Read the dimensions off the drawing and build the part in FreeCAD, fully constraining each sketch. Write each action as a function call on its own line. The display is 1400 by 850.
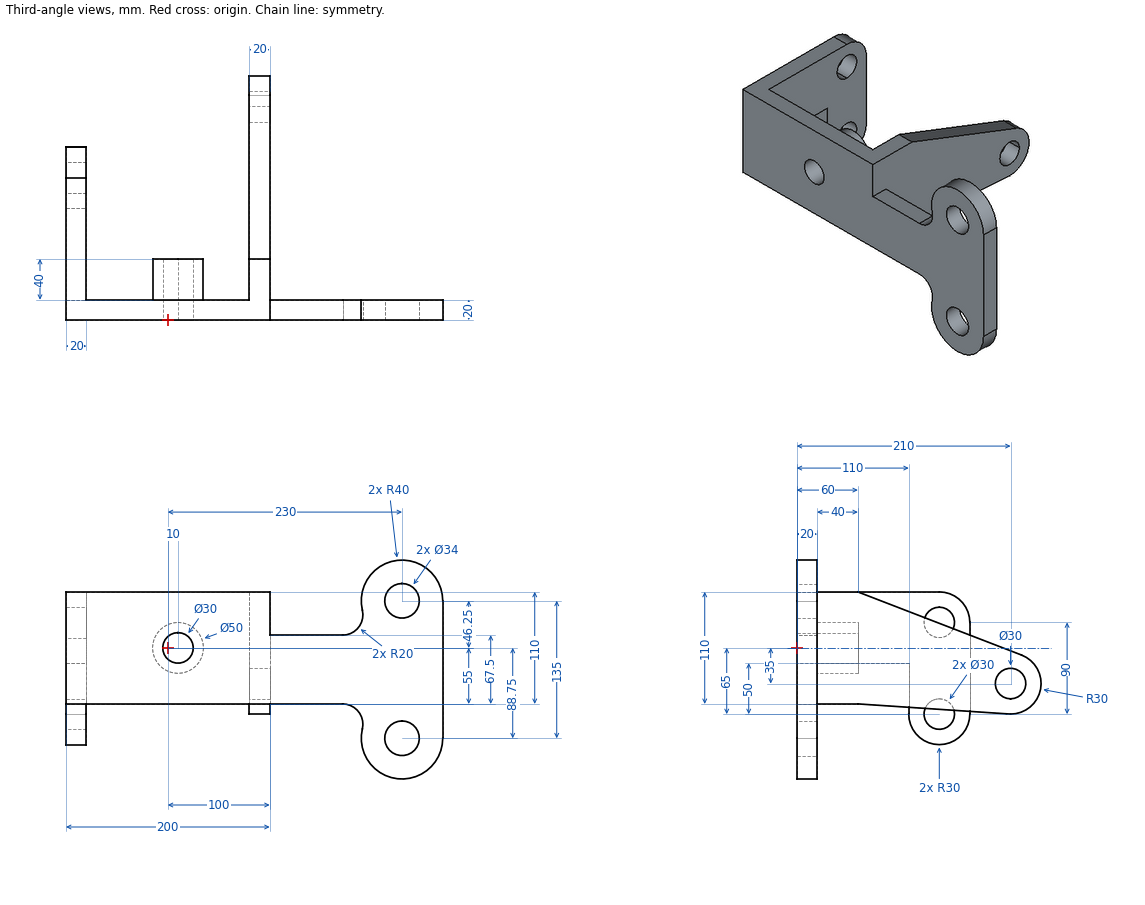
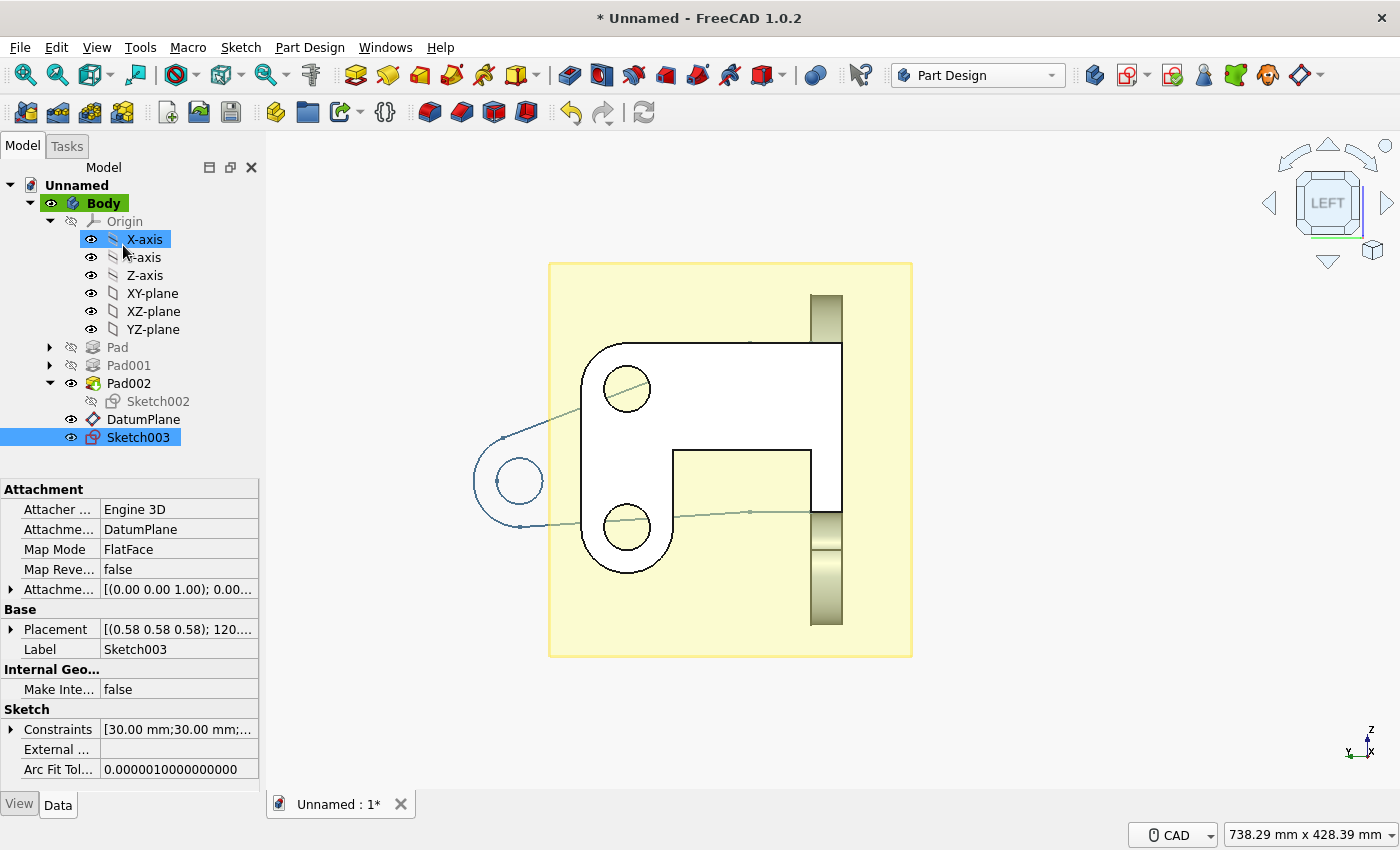
click(356, 76)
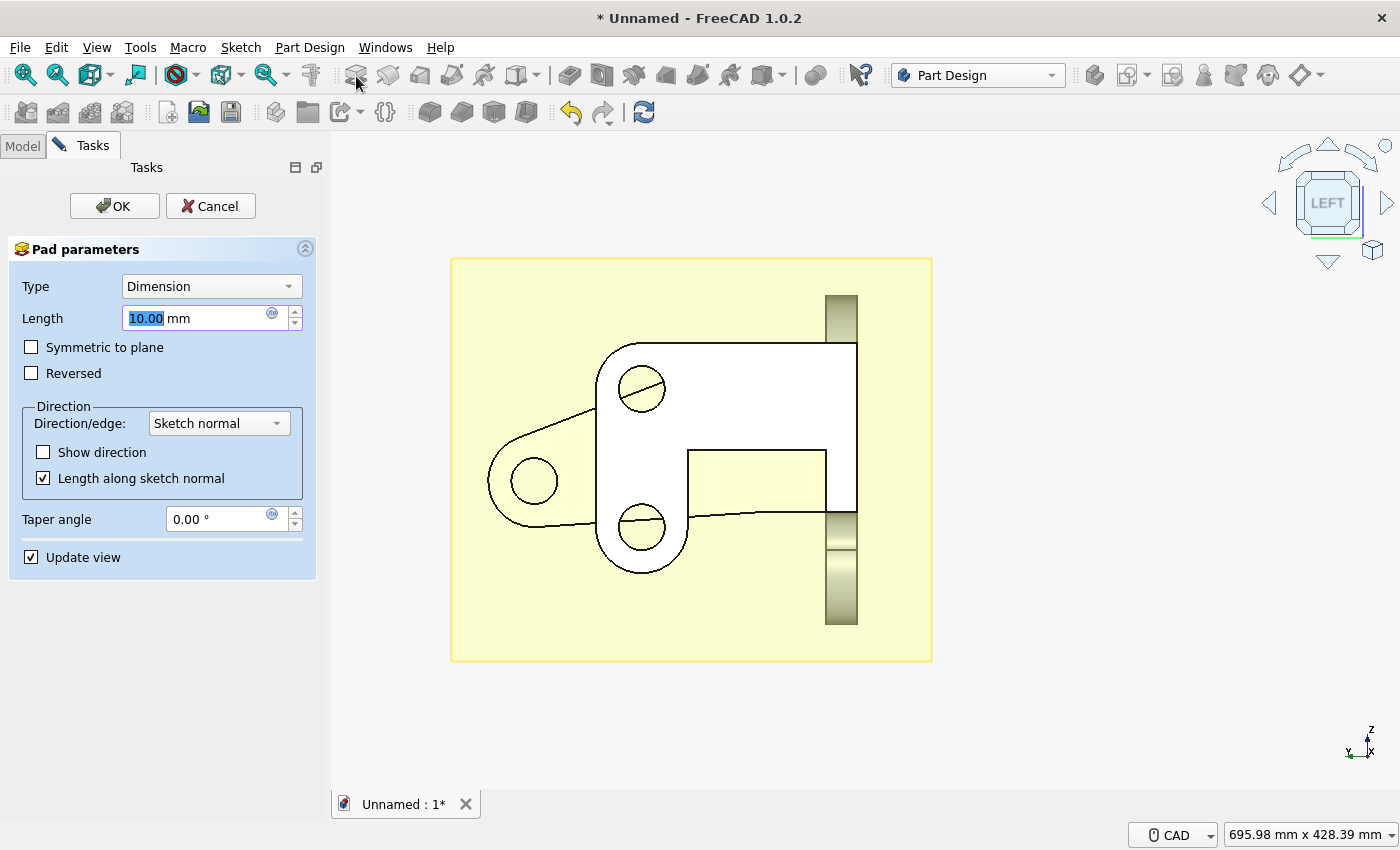
text(20)
key(Tab)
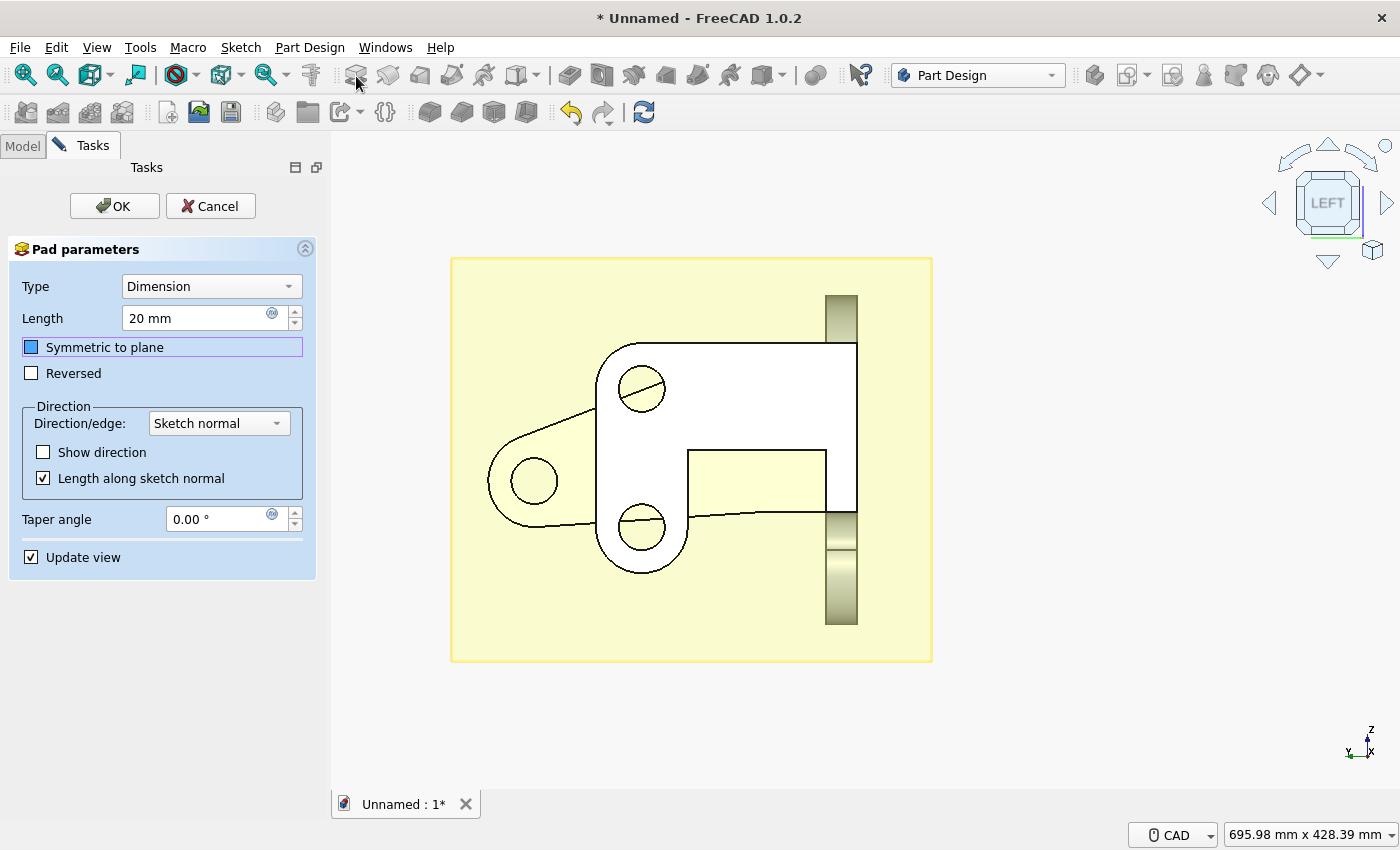
click(30, 373)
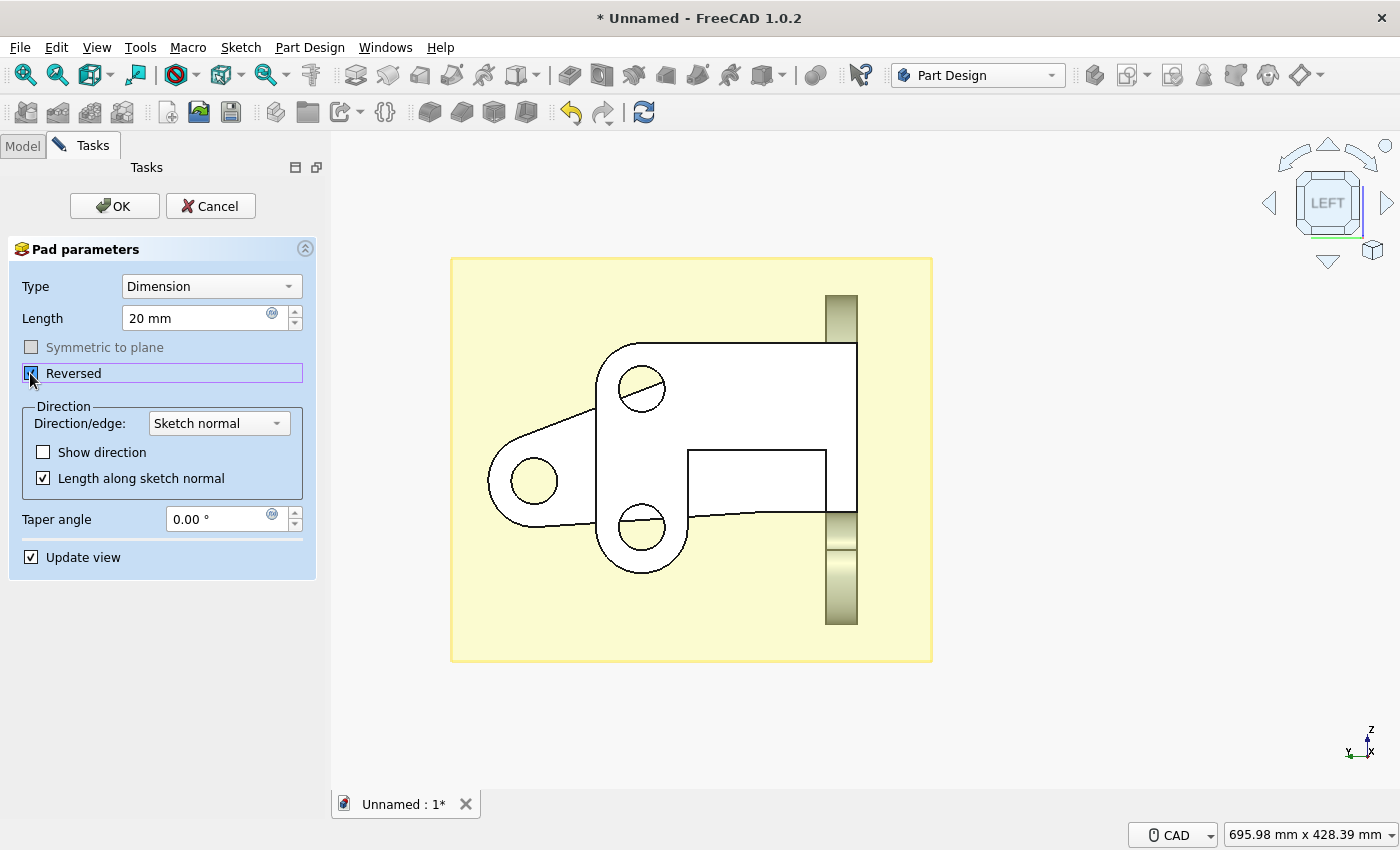
click(115, 206)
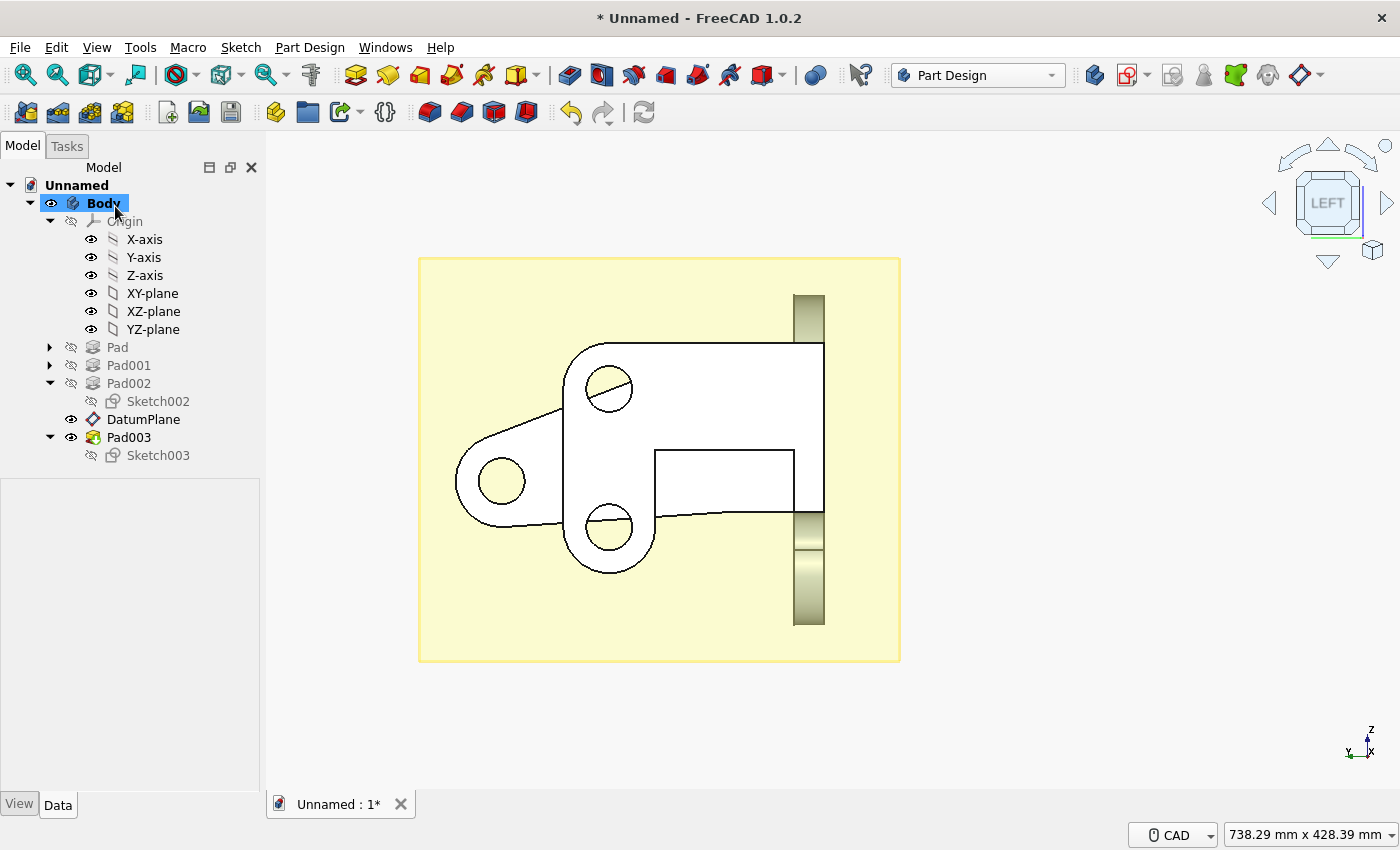
click(116, 419)
key(space)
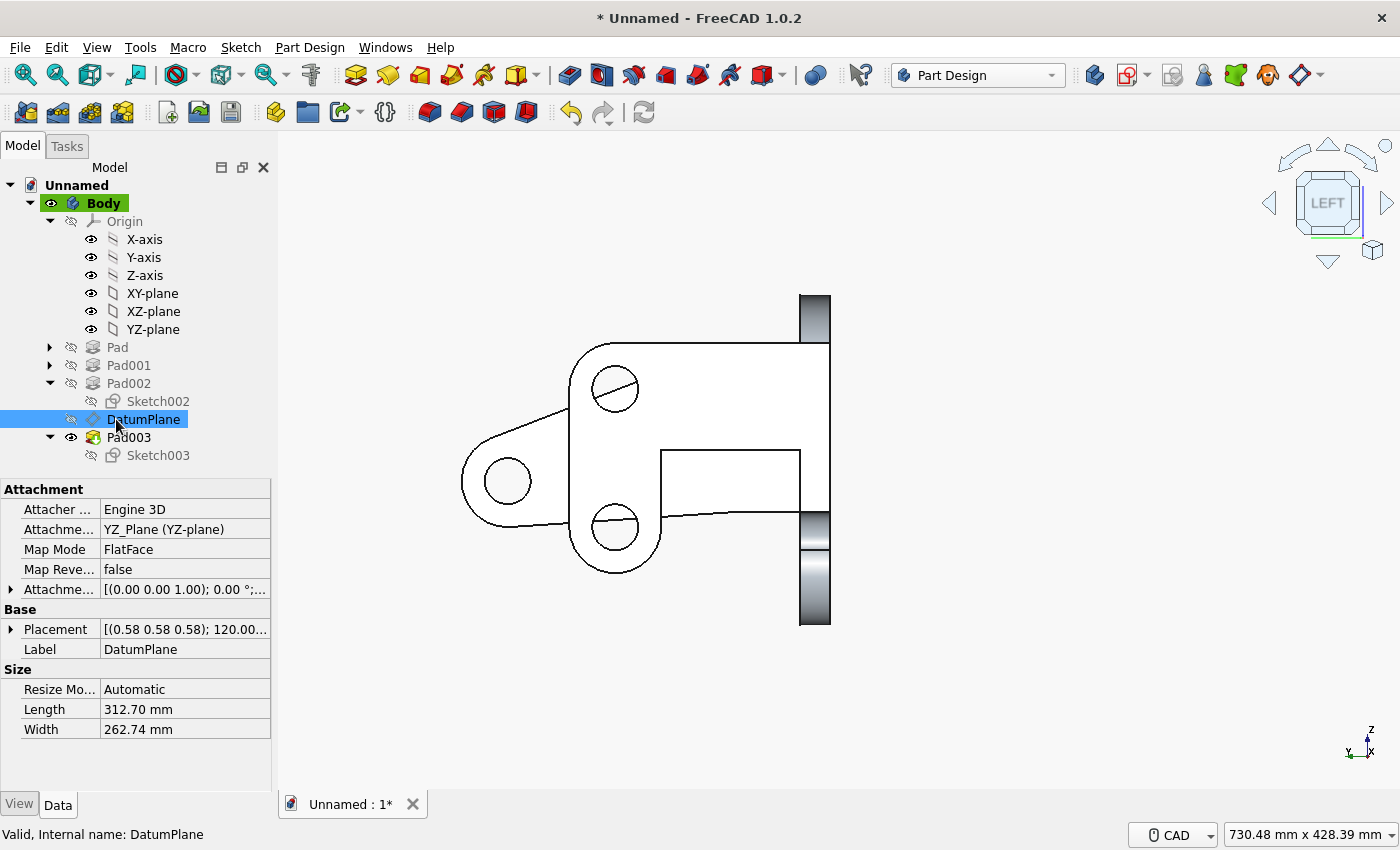
key(4)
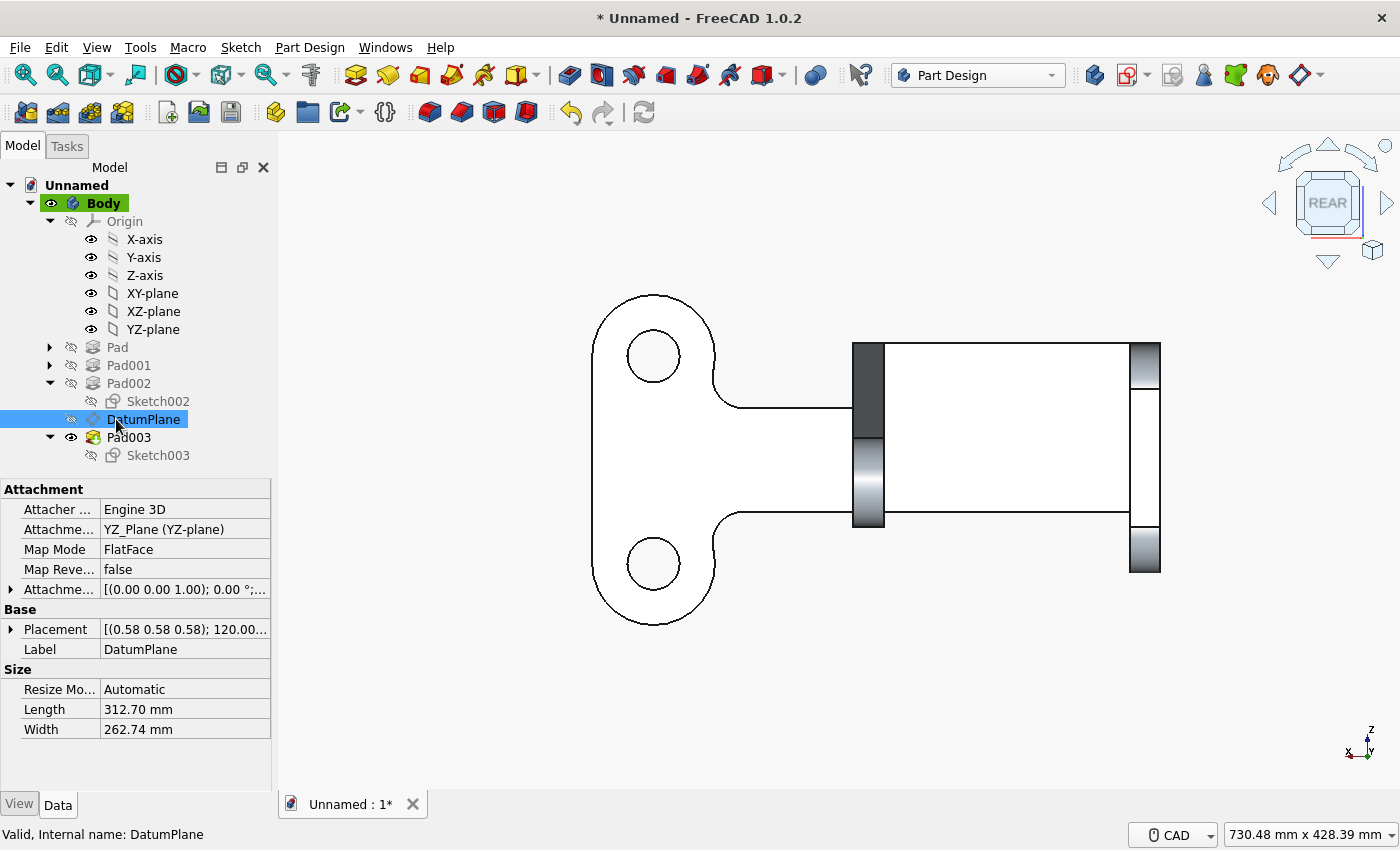
click(685, 459)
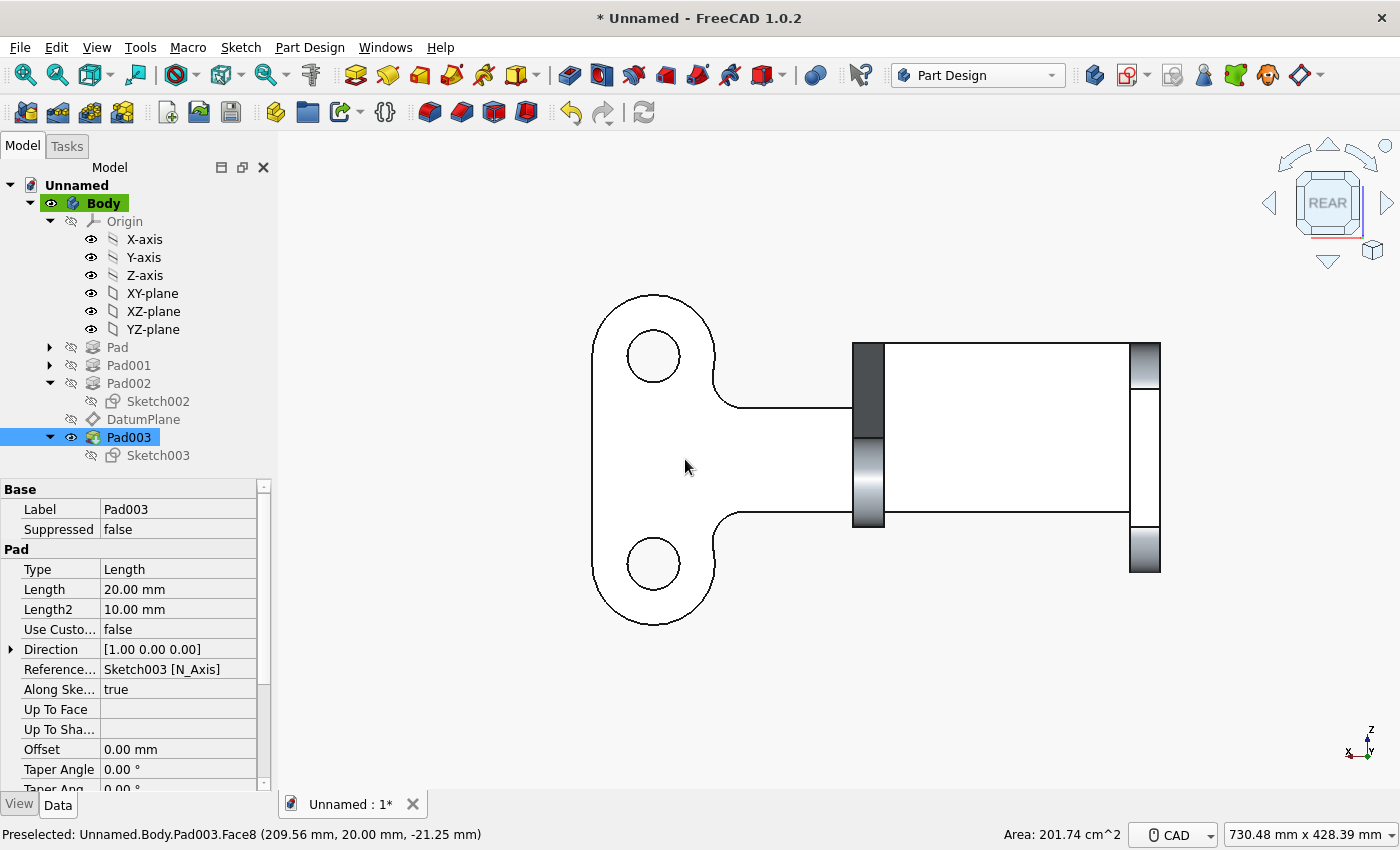
click(1128, 76)